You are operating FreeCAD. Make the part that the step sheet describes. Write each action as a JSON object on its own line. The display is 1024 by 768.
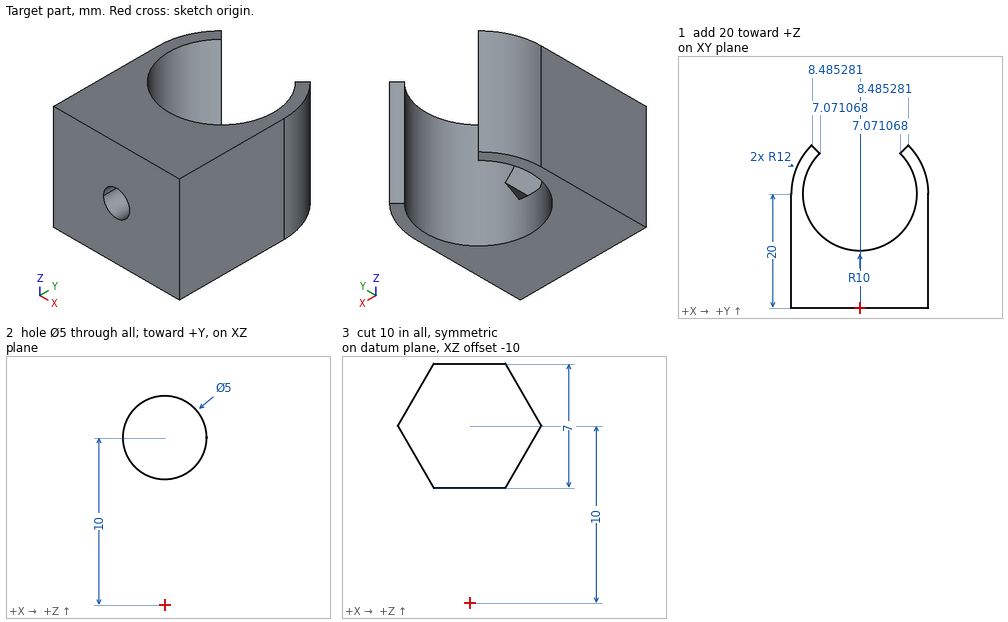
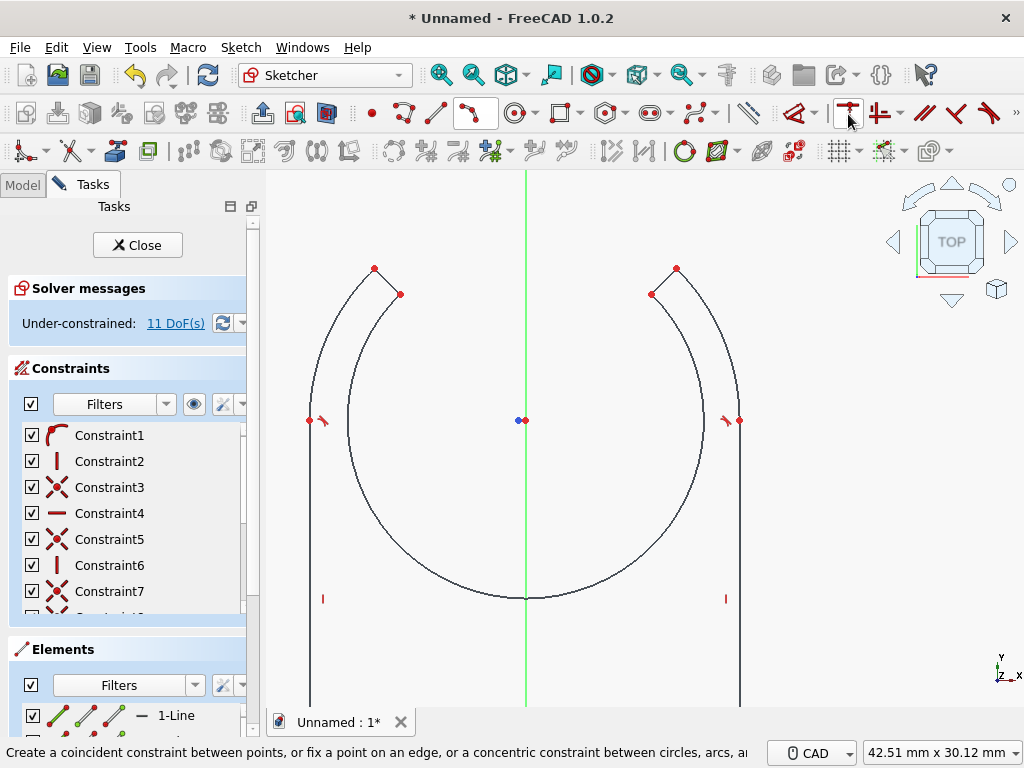
{"action": "left_click", "coordinate": [734, 370]}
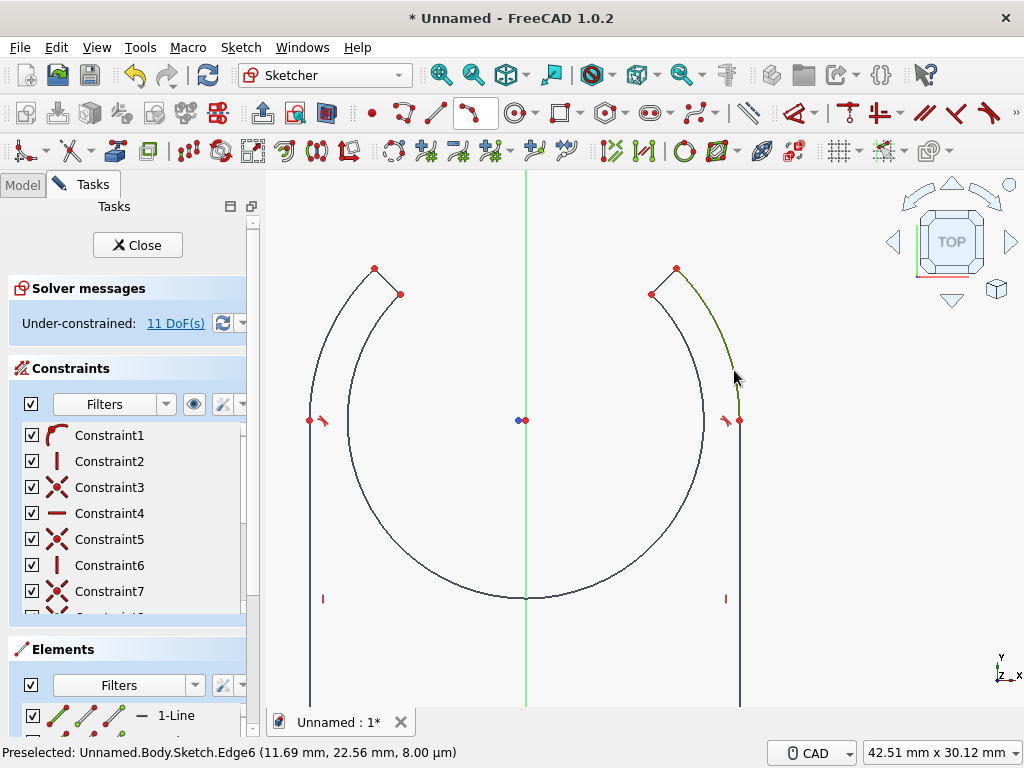
{"action": "left_click", "coordinate": [343, 308]}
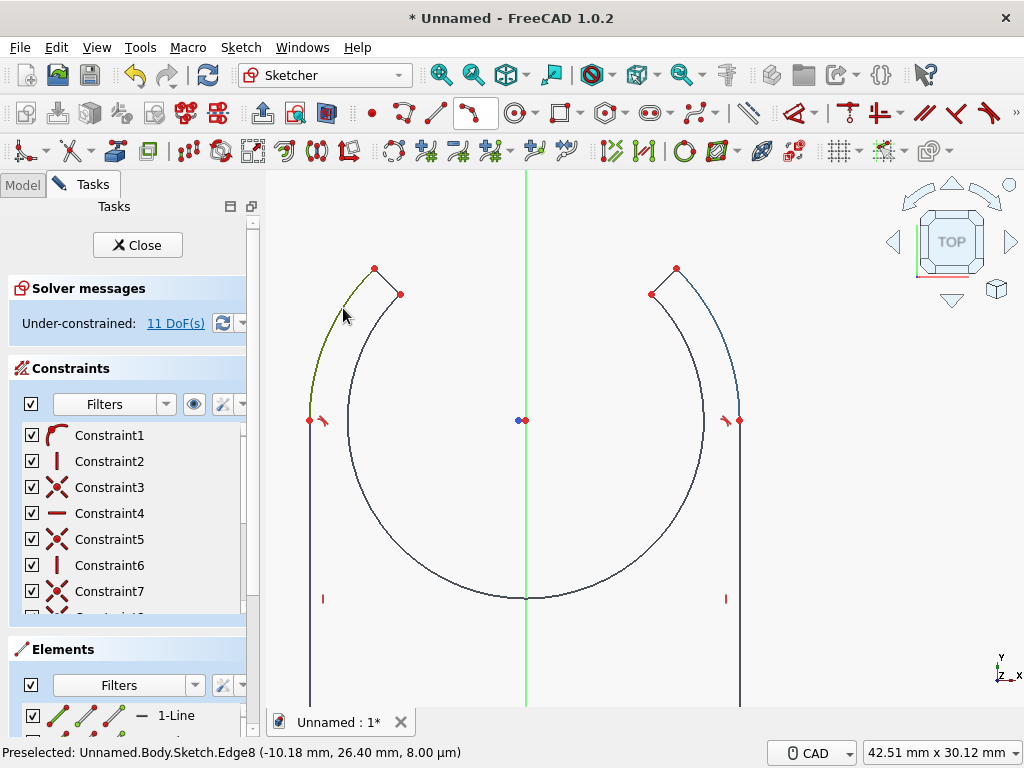
{"action": "left_click", "coordinate": [848, 114]}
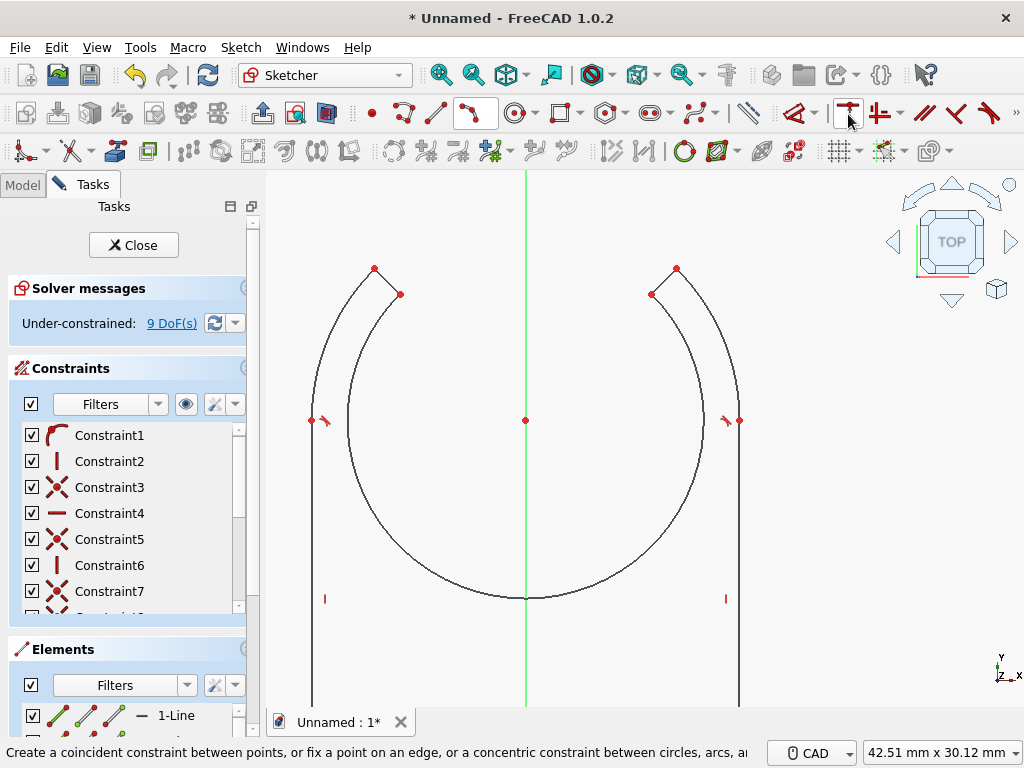
{"action": "left_click", "coordinate": [734, 370]}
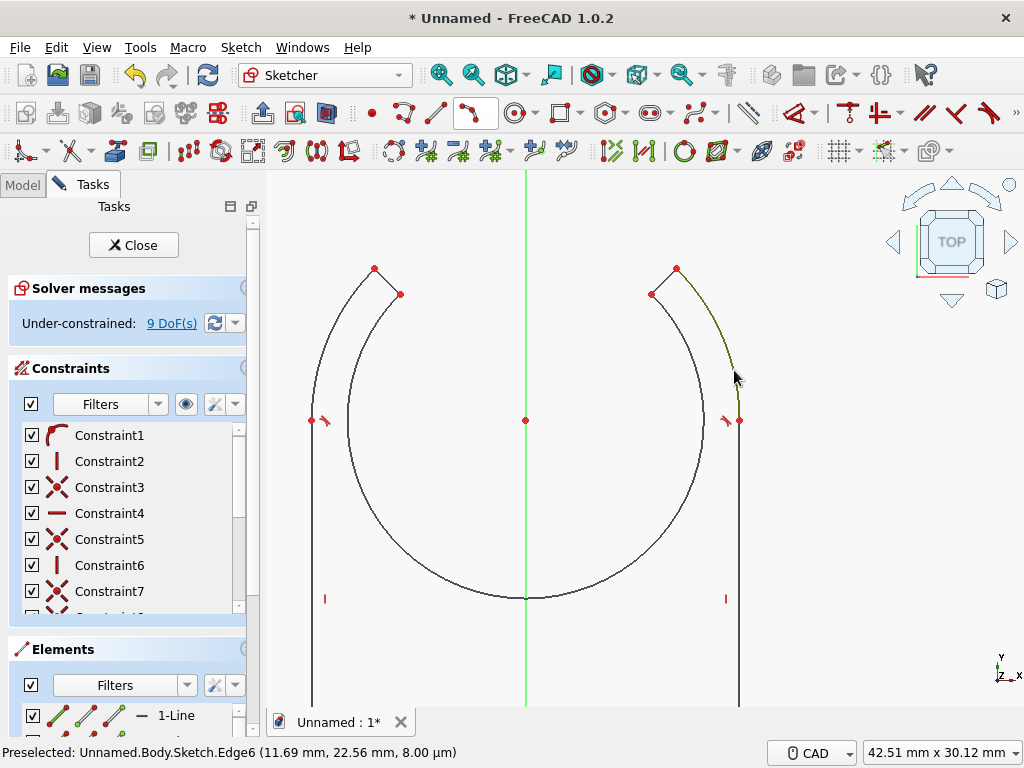
{"action": "left_click", "coordinate": [344, 308]}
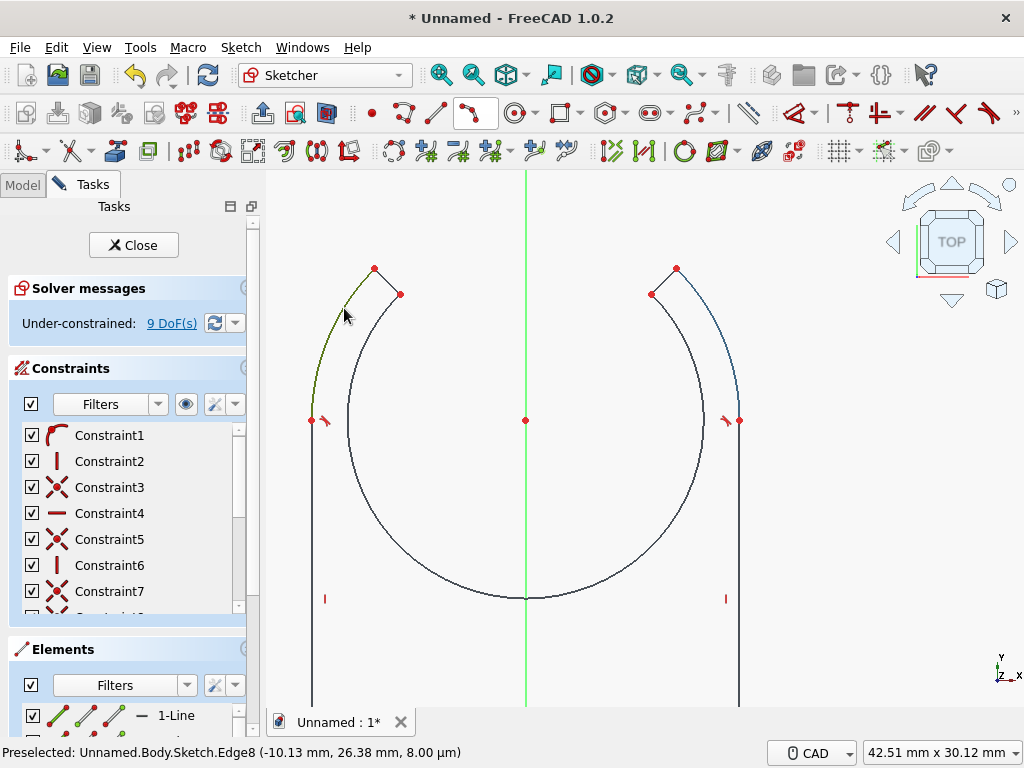
{"action": "key", "text": "e"}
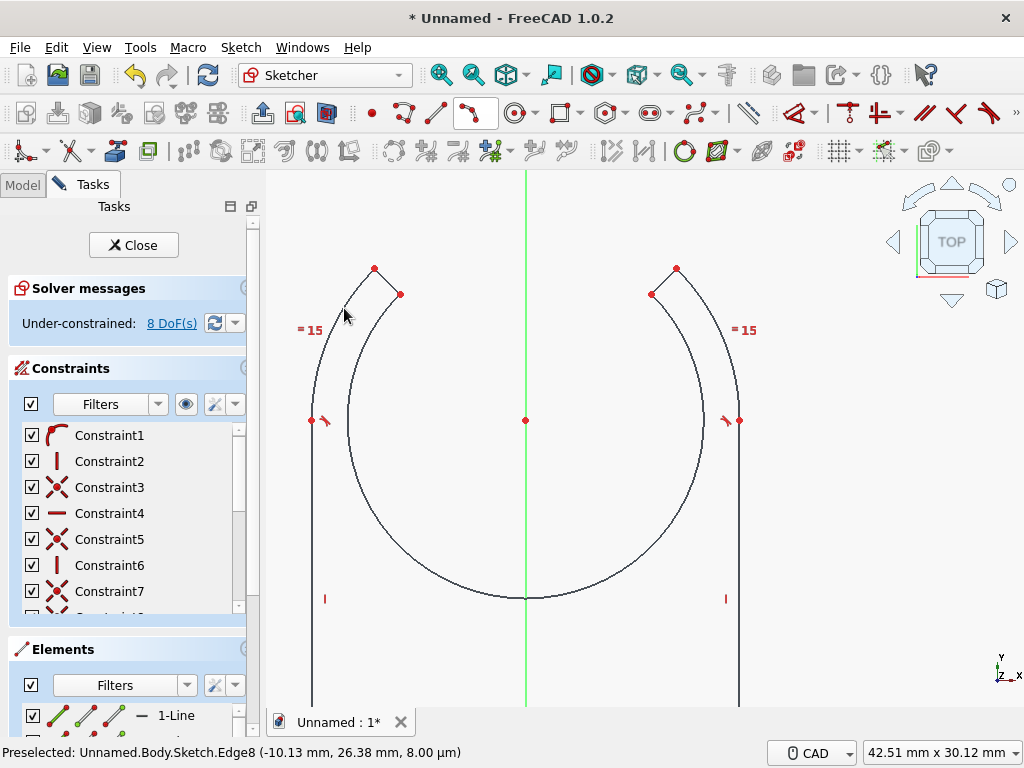
{"action": "left_click", "coordinate": [526, 420]}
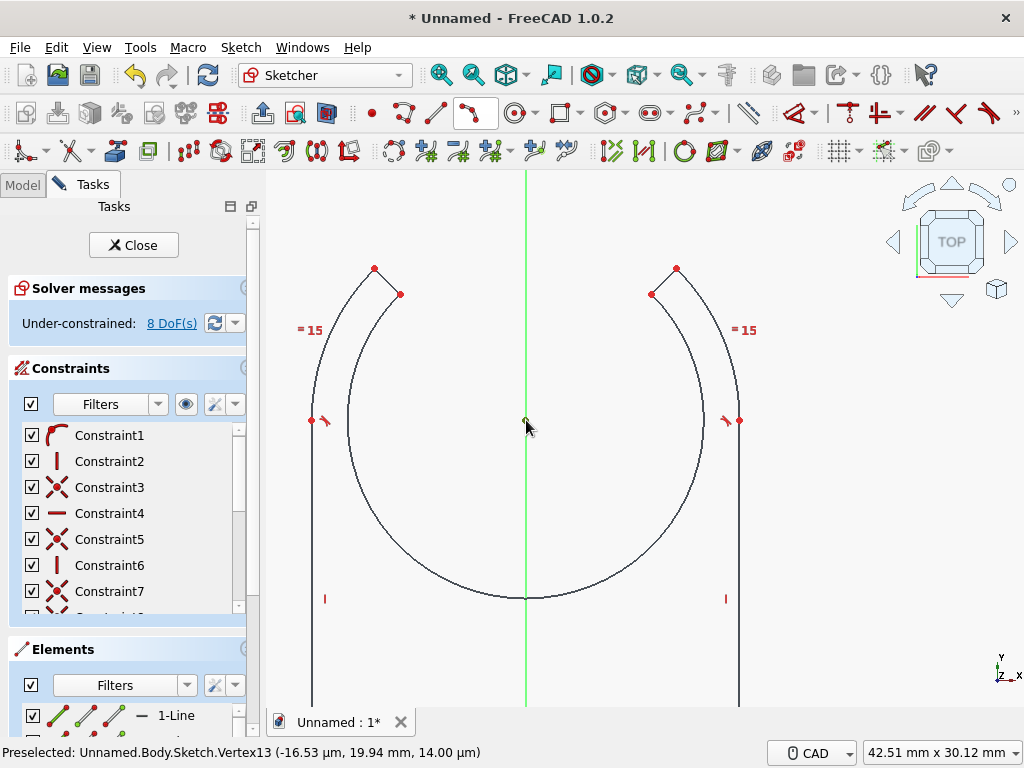
{"action": "left_click", "coordinate": [526, 645]}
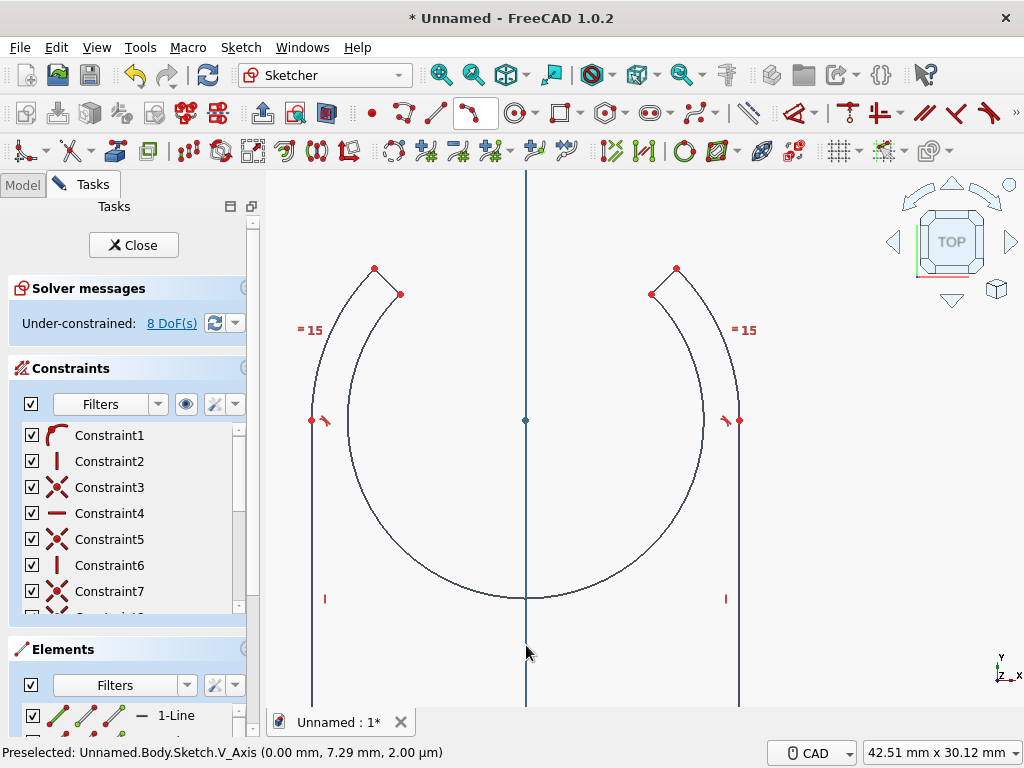
{"action": "left_click", "coordinate": [848, 114]}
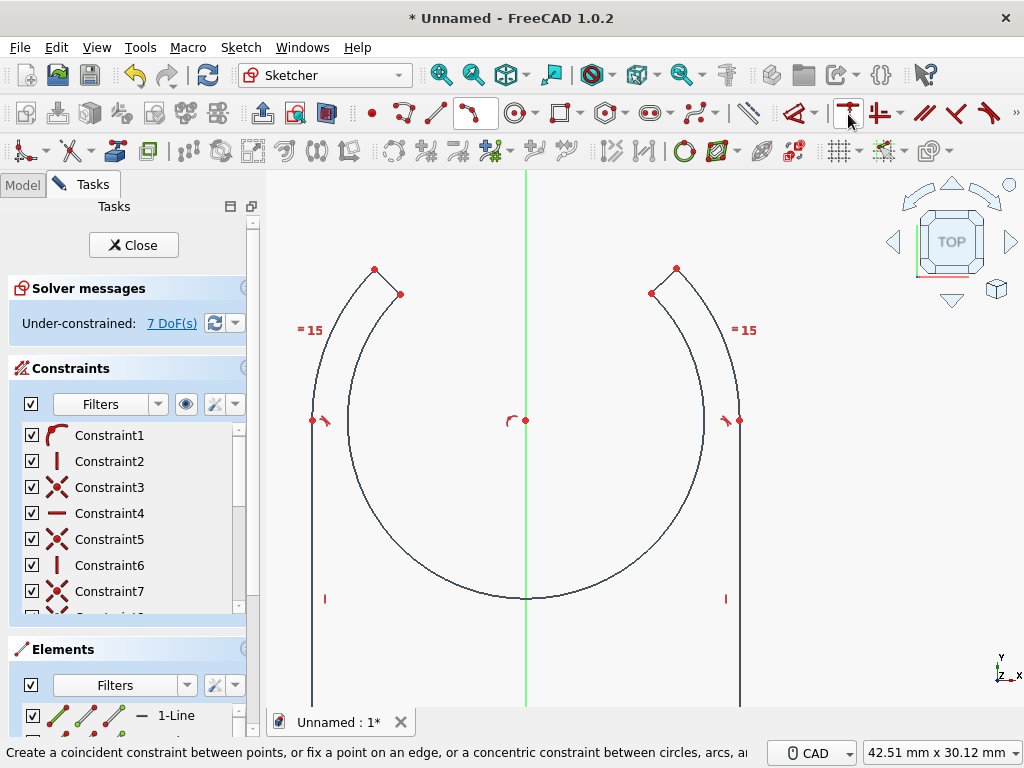
{"action": "left_click", "coordinate": [794, 114]}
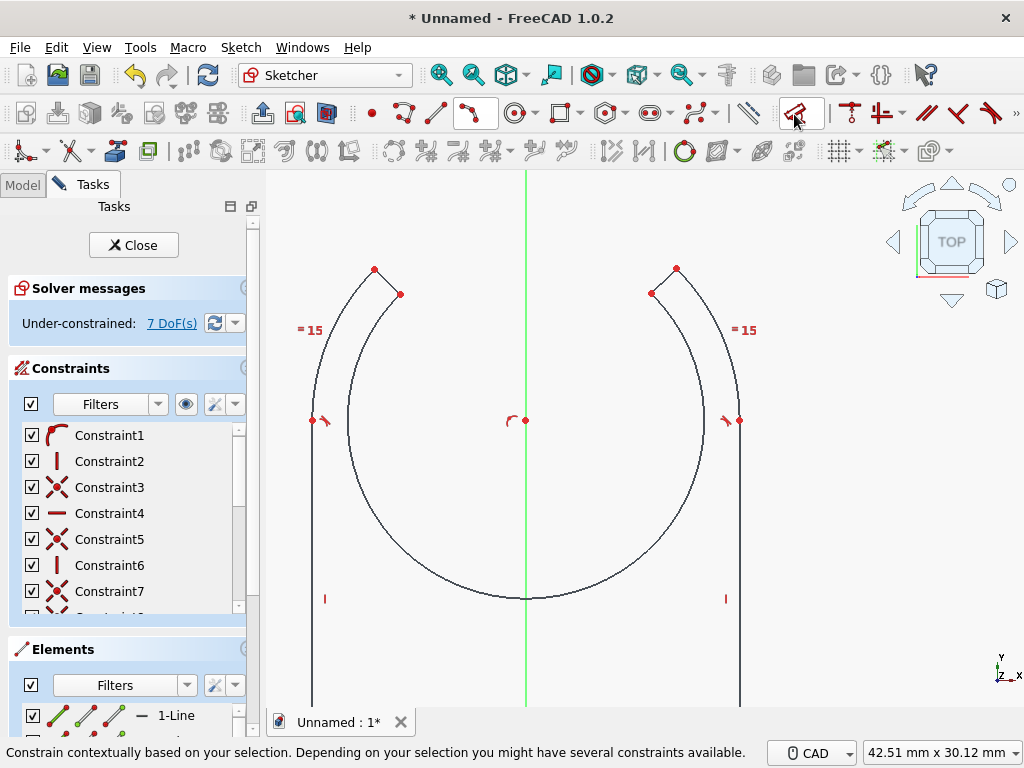
{"action": "left_click", "coordinate": [734, 370]}
{"action": "left_click", "coordinate": [765, 362]}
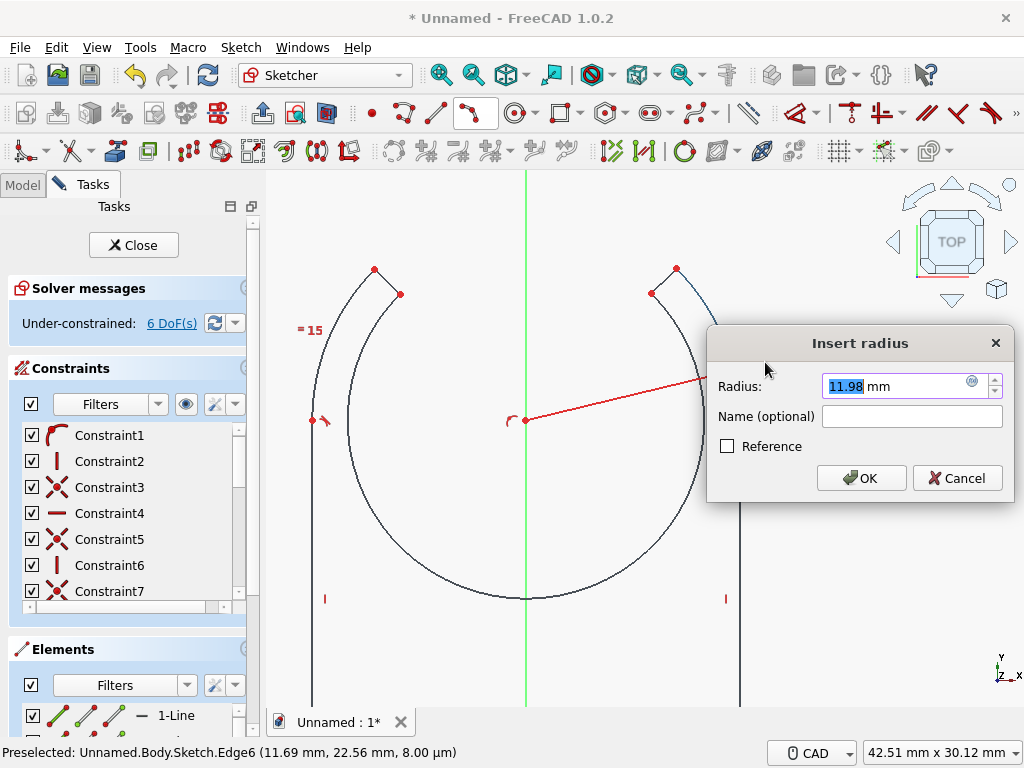
{"action": "type", "text": "12"}
{"action": "key", "text": "Return"}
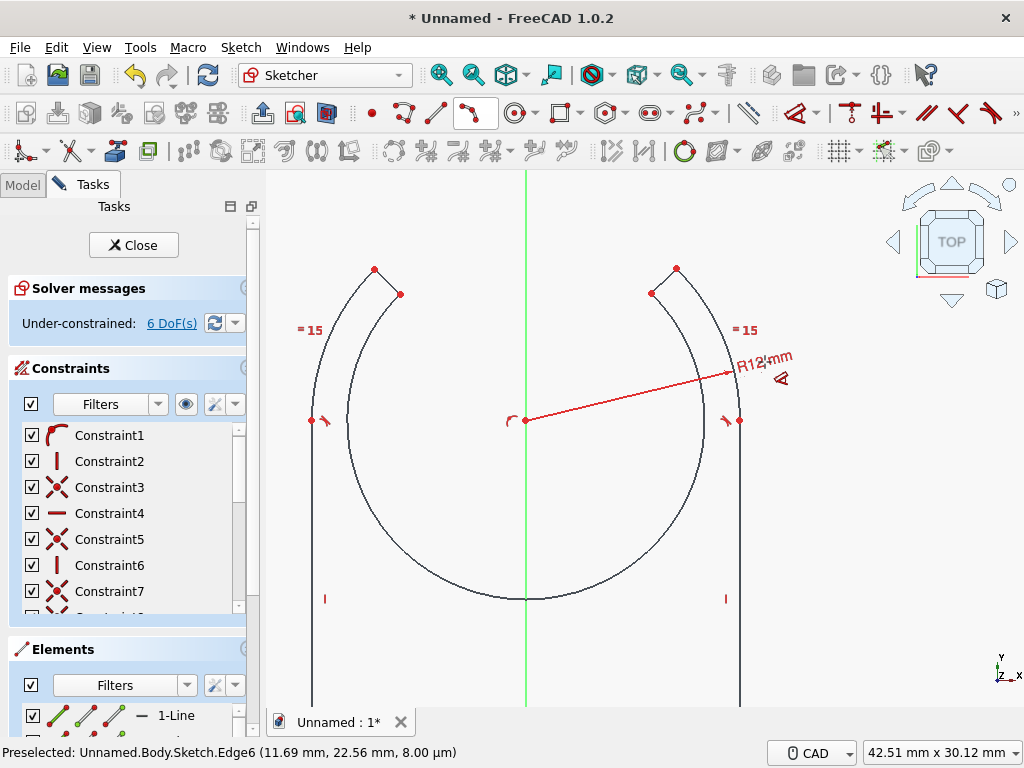
{"action": "left_click", "coordinate": [381, 526]}
{"action": "left_click", "coordinate": [355, 545]}